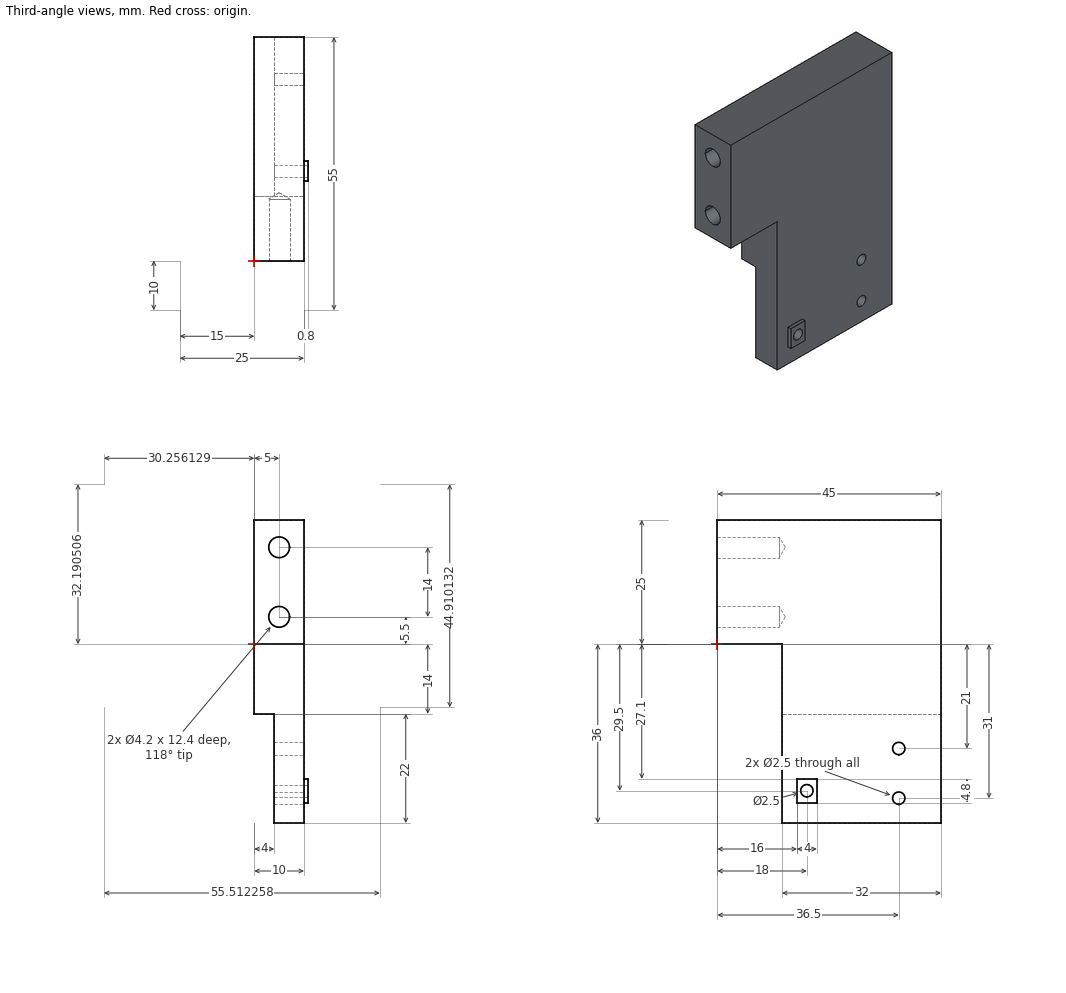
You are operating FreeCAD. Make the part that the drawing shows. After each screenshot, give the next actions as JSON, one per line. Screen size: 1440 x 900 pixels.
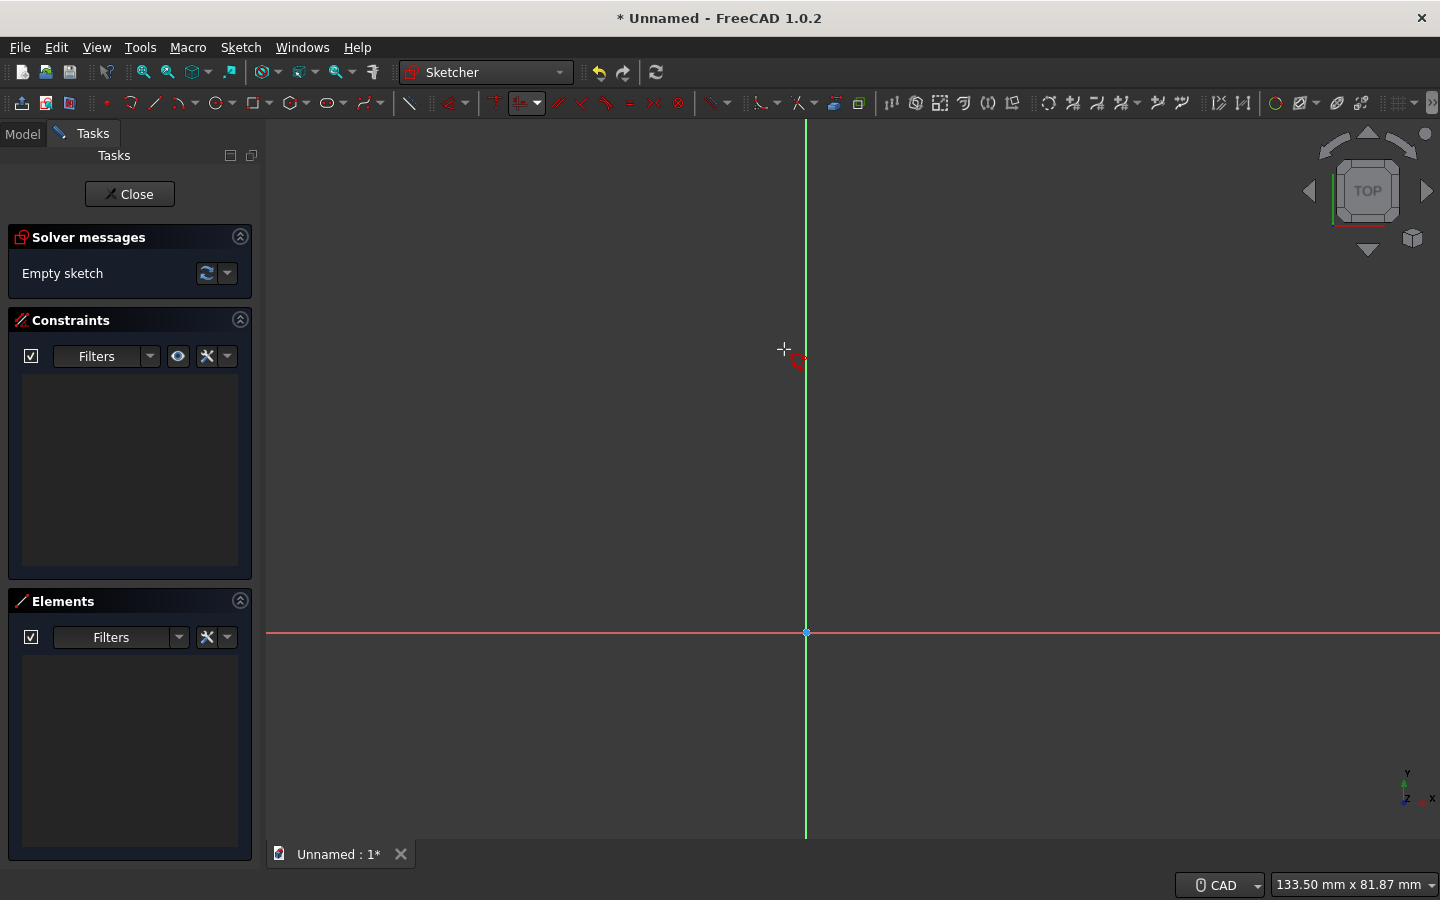
{"action": "left_click", "coordinate": [806, 633]}
{"action": "left_click", "coordinate": [675, 624]}
{"action": "left_click", "coordinate": [675, 721]}
{"action": "left_click", "coordinate": [894, 721]}
{"action": "left_click", "coordinate": [894, 237]}
{"action": "left_click", "coordinate": [797, 237]}
{"action": "left_click", "coordinate": [806, 633]}
{"action": "key", "text": "Escape"}
{"action": "key", "text": "Escape"}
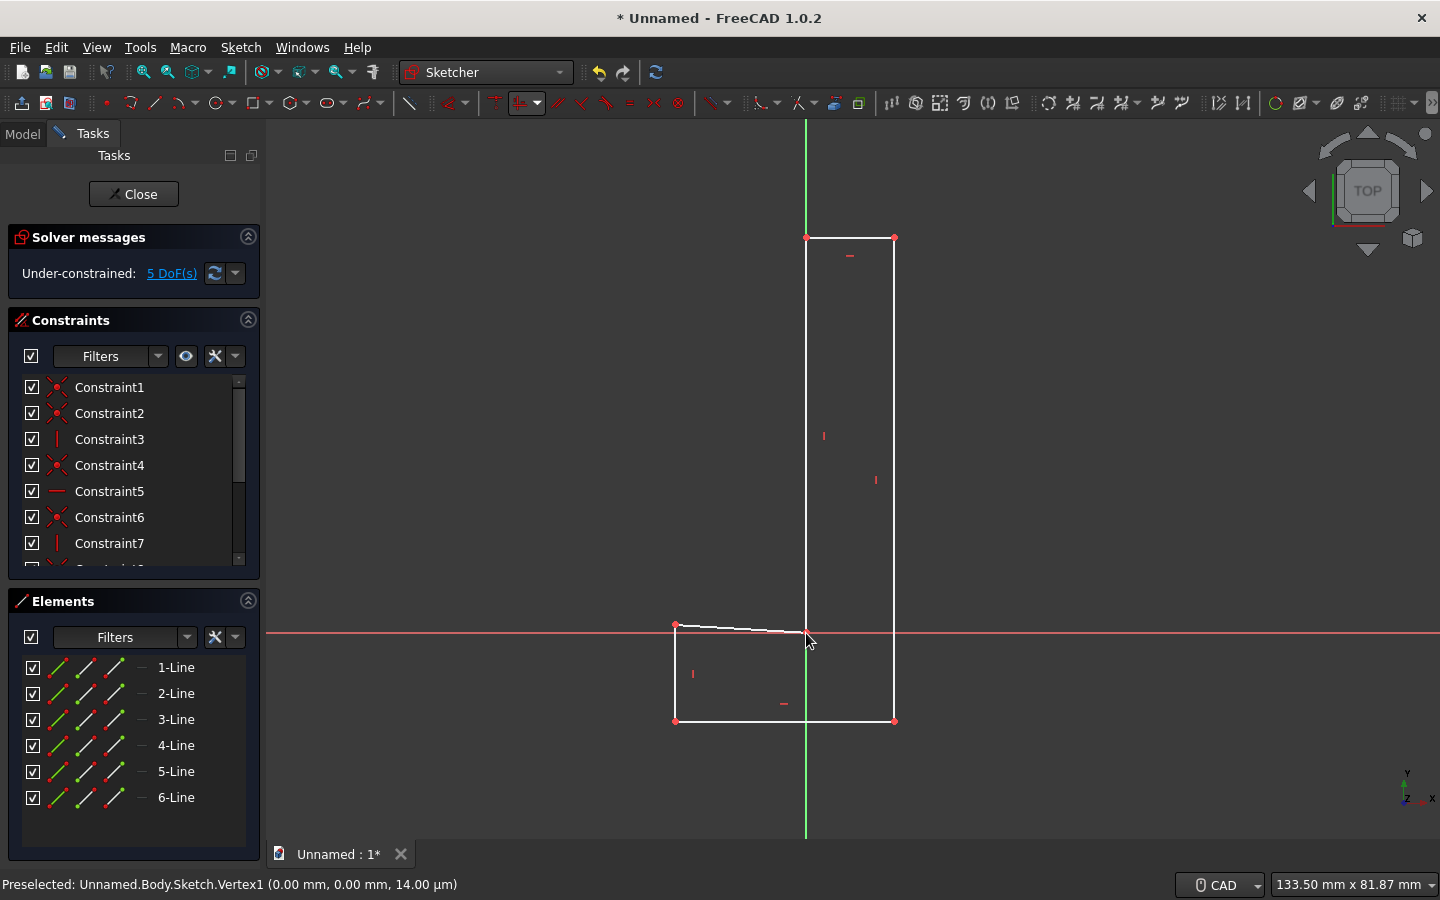
{"action": "left_click", "coordinate": [767, 630]}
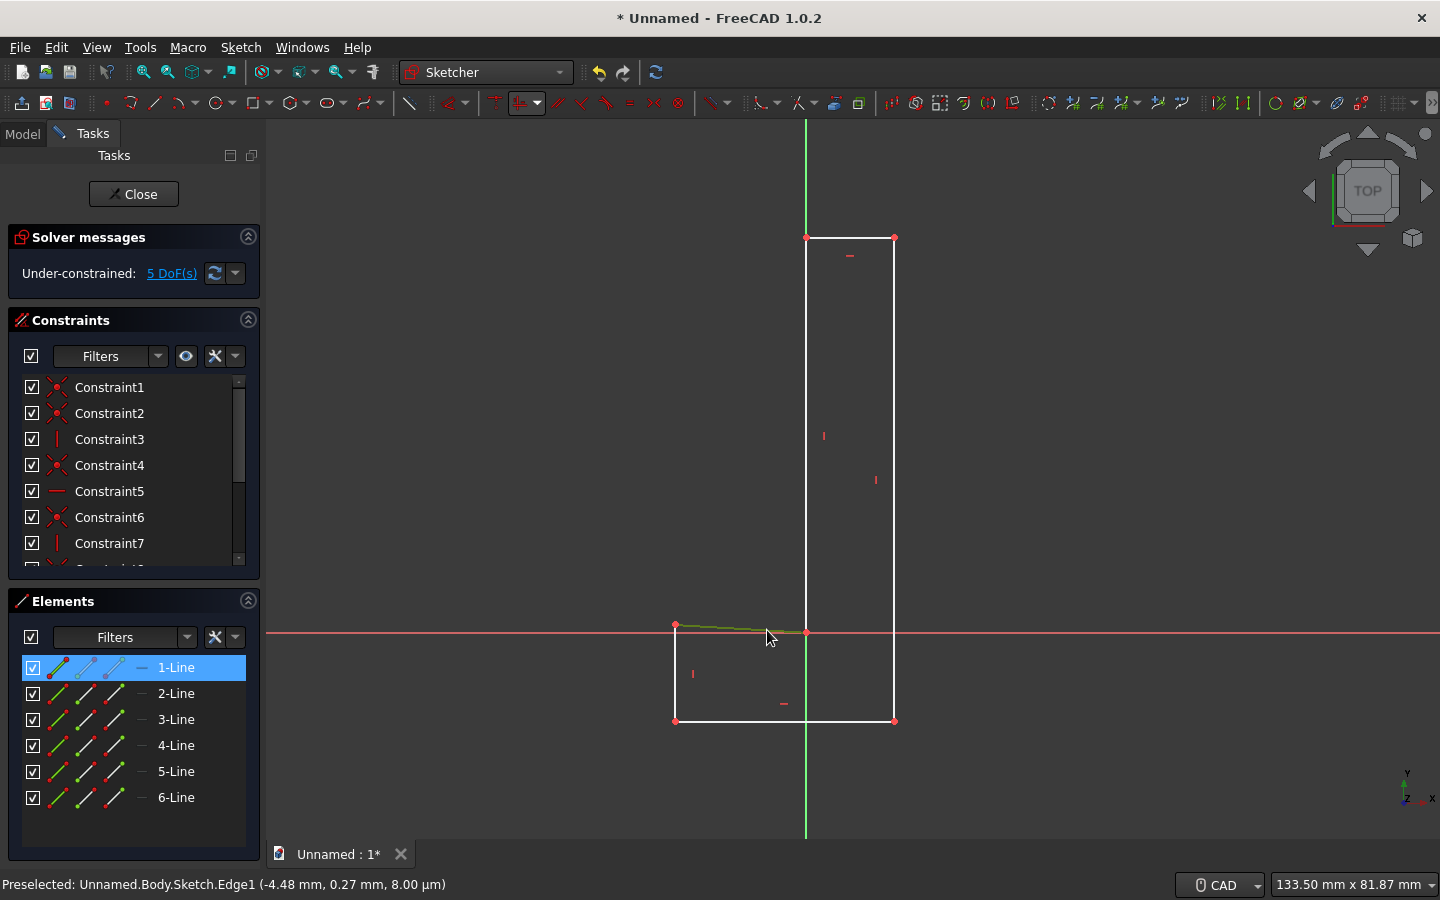
{"action": "key", "text": "h"}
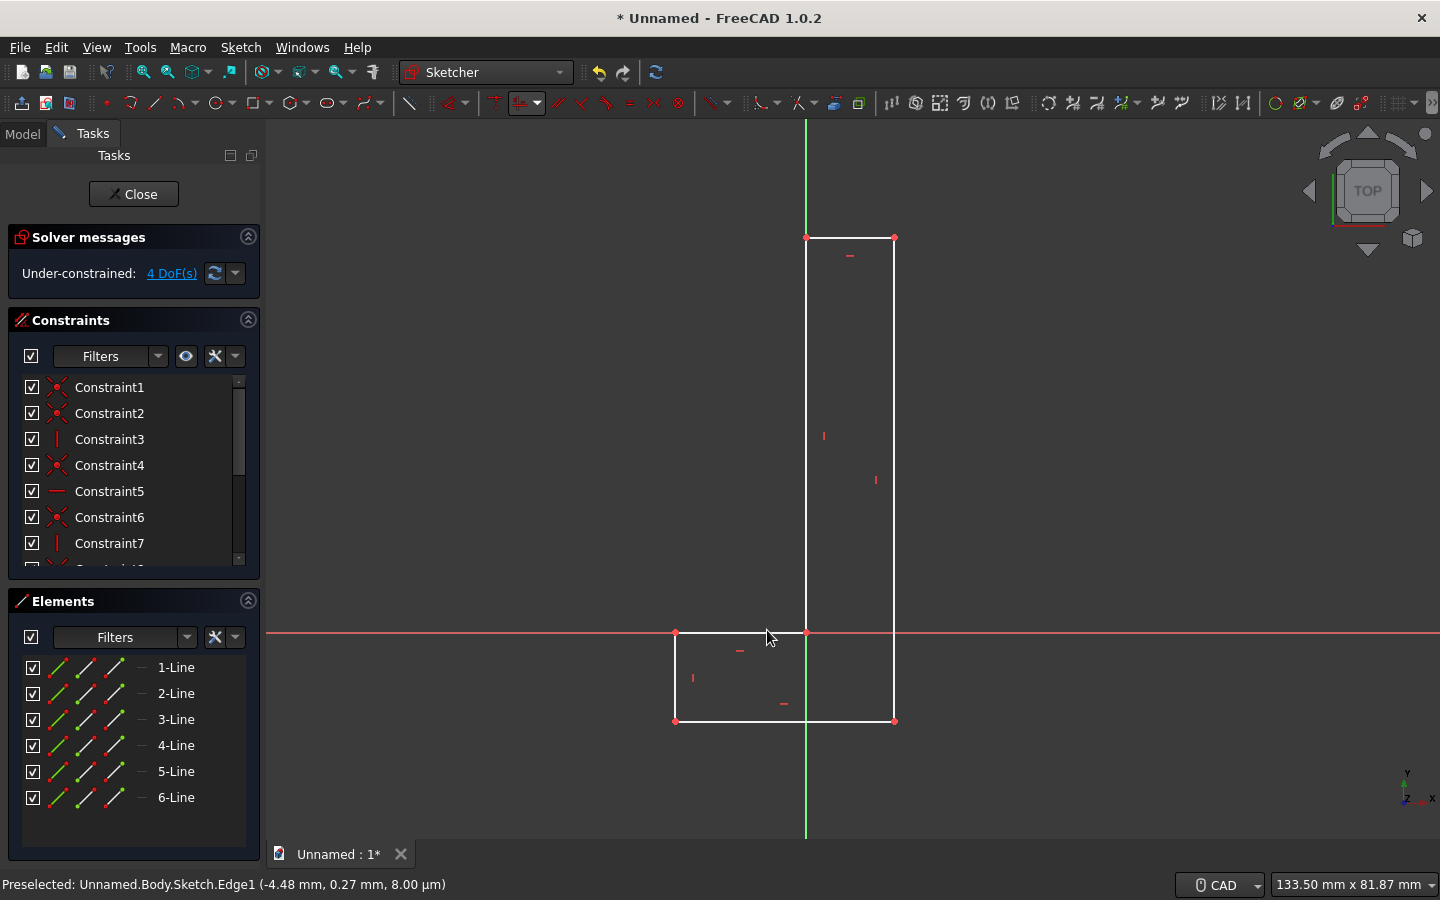
{"action": "left_click", "coordinate": [767, 633]}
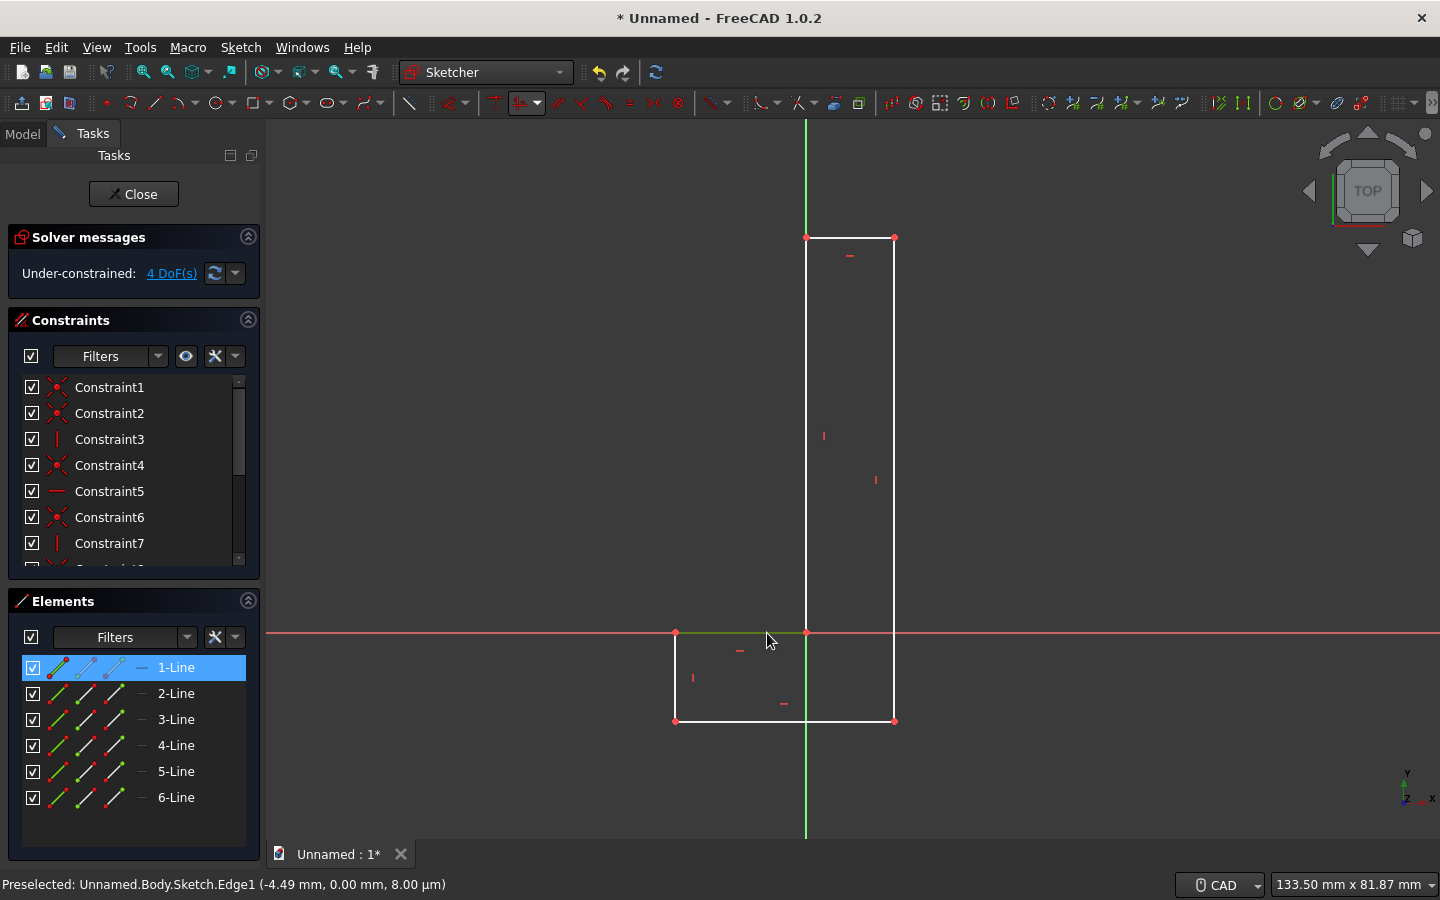
{"action": "key", "text": "l"}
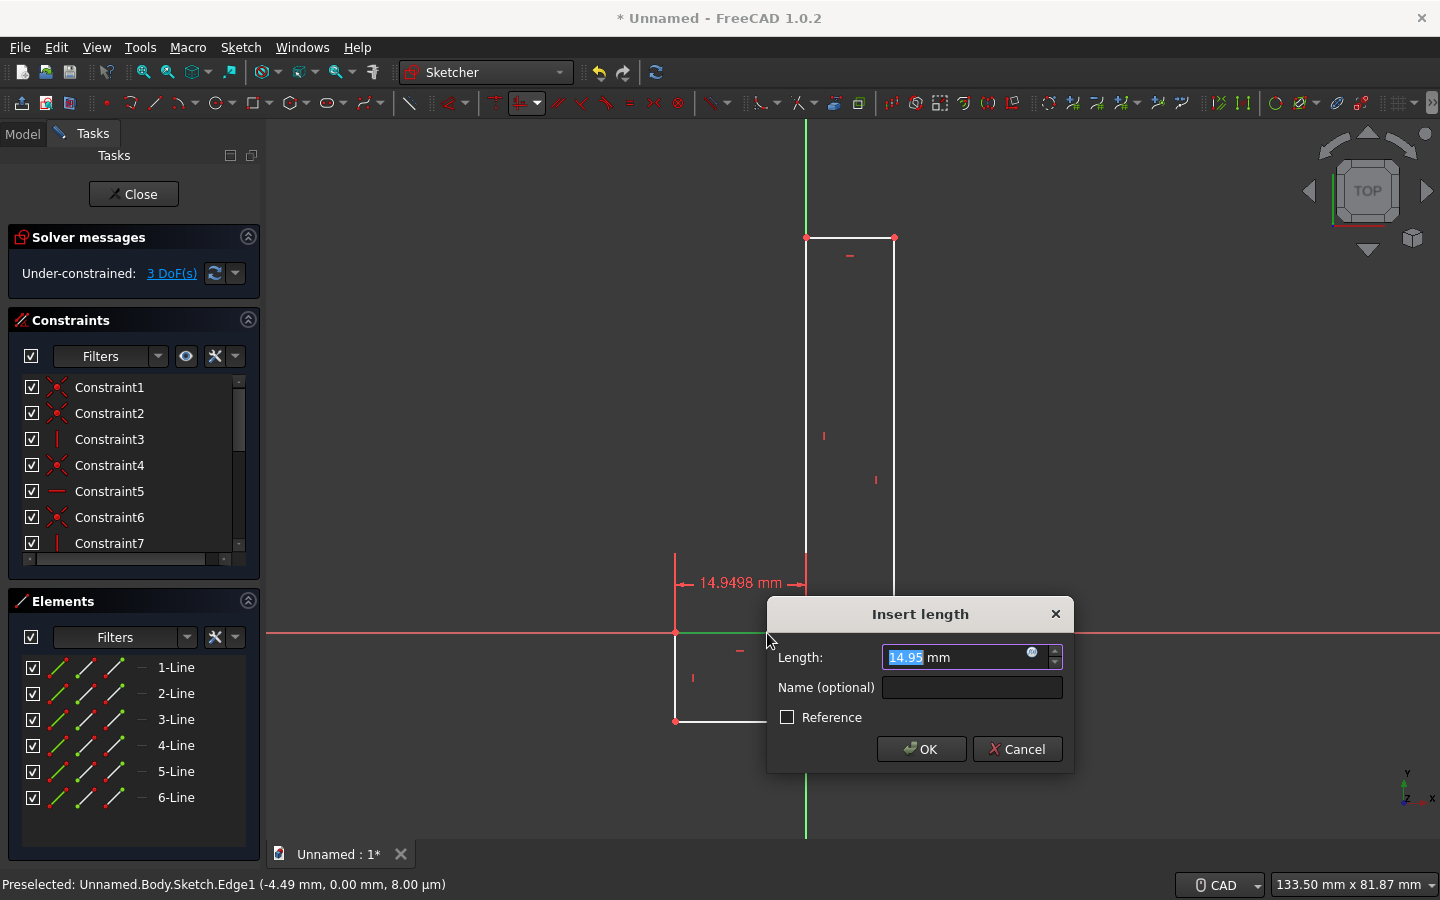
{"action": "type", "text": "15"}
{"action": "key", "text": "Return"}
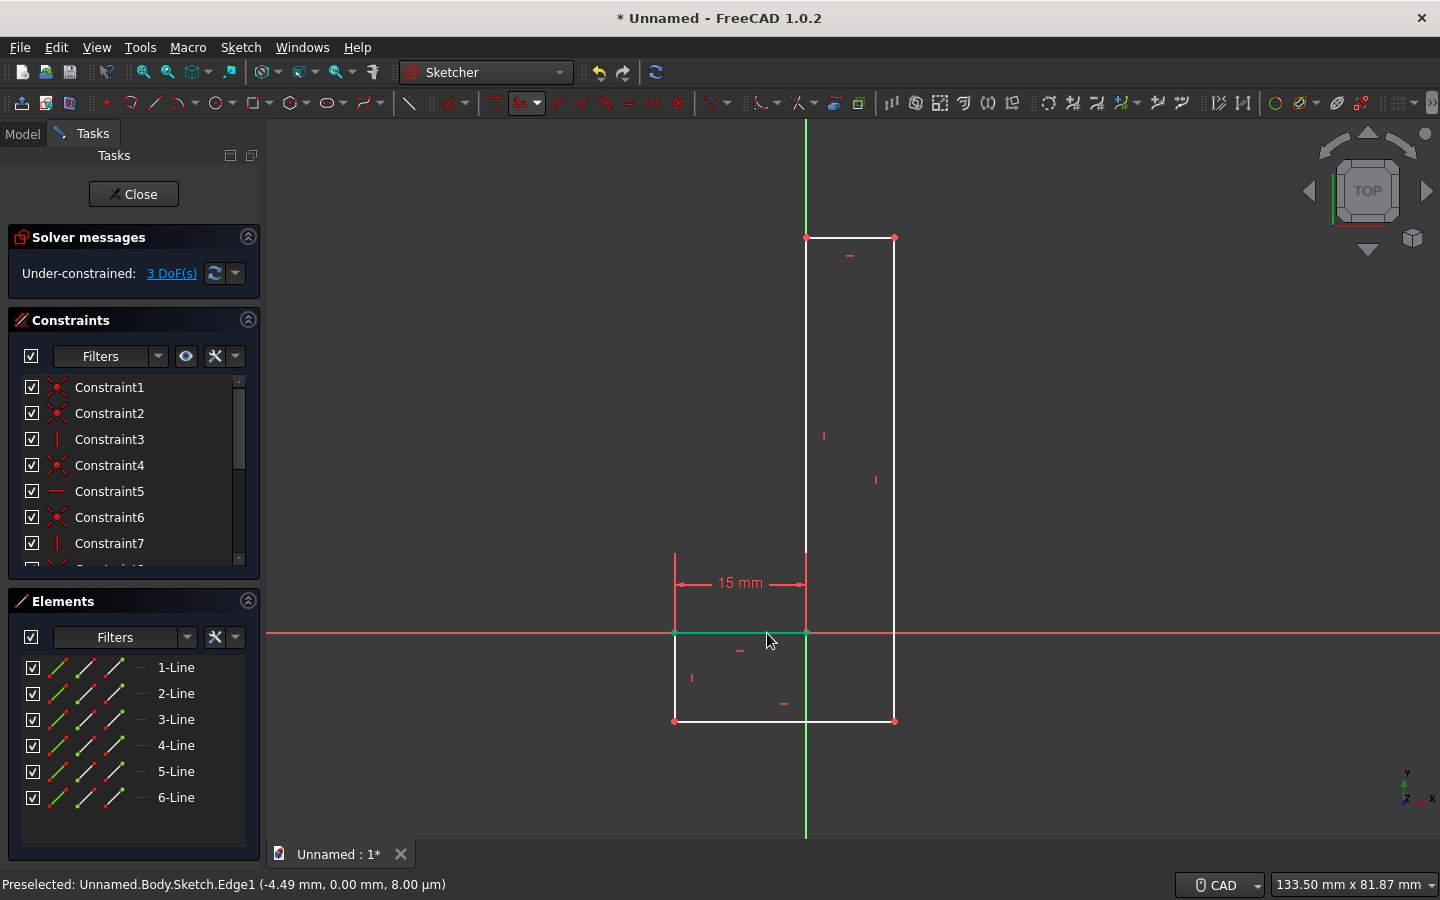
{"action": "left_click", "coordinate": [675, 660]}